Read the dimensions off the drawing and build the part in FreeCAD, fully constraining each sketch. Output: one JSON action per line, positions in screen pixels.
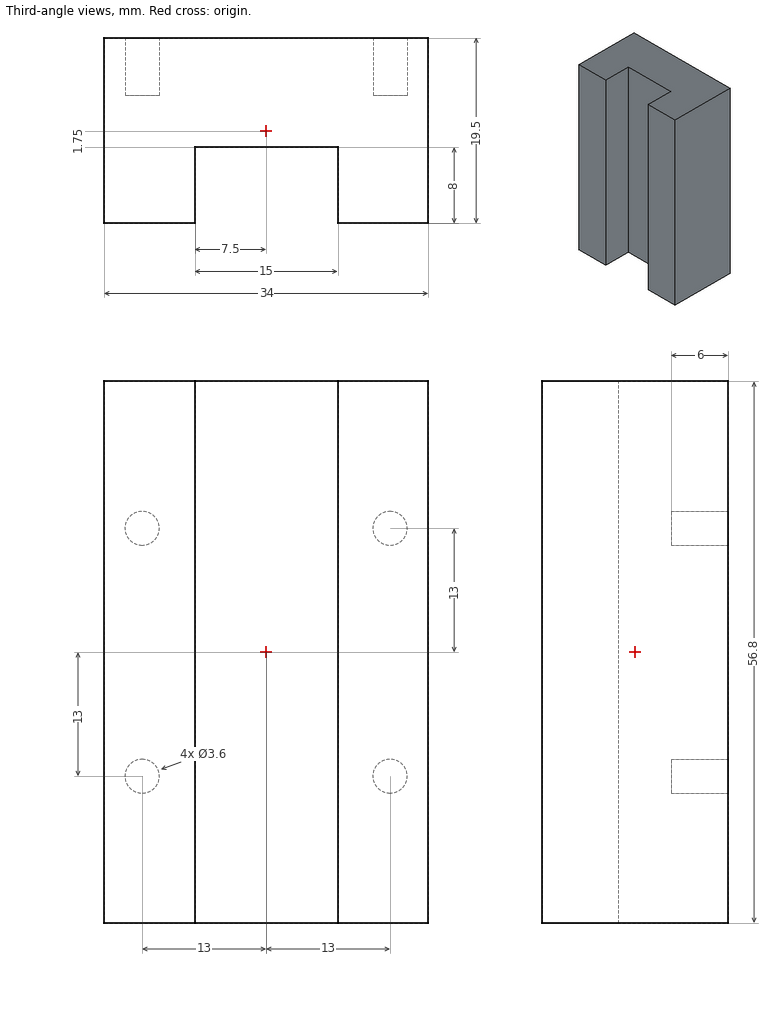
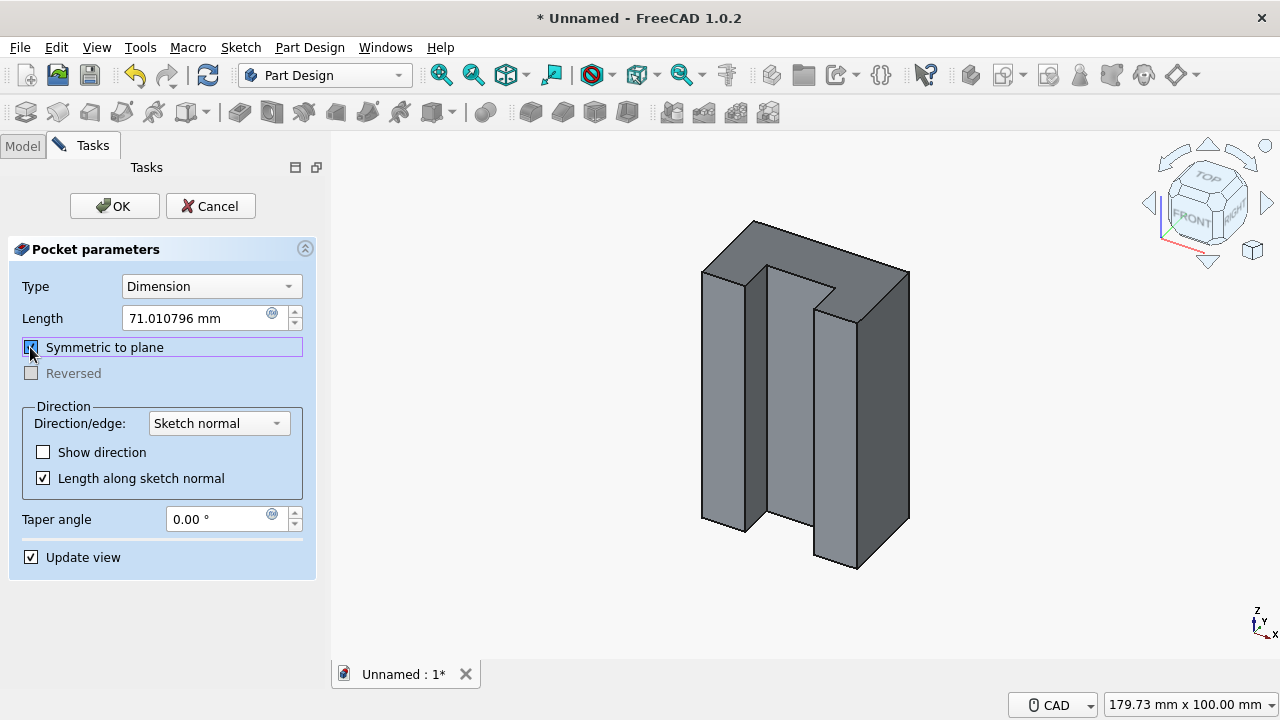
{"action": "left_click", "coordinate": [115, 206]}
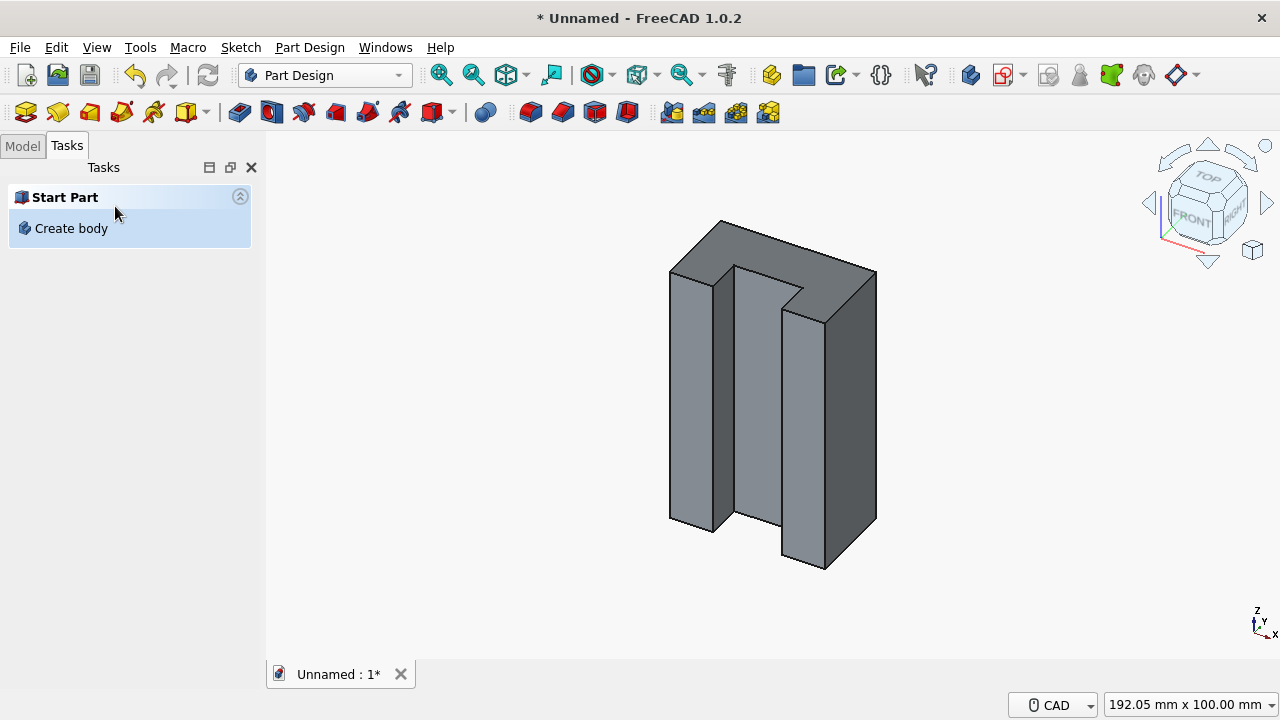
{"action": "key", "text": "4"}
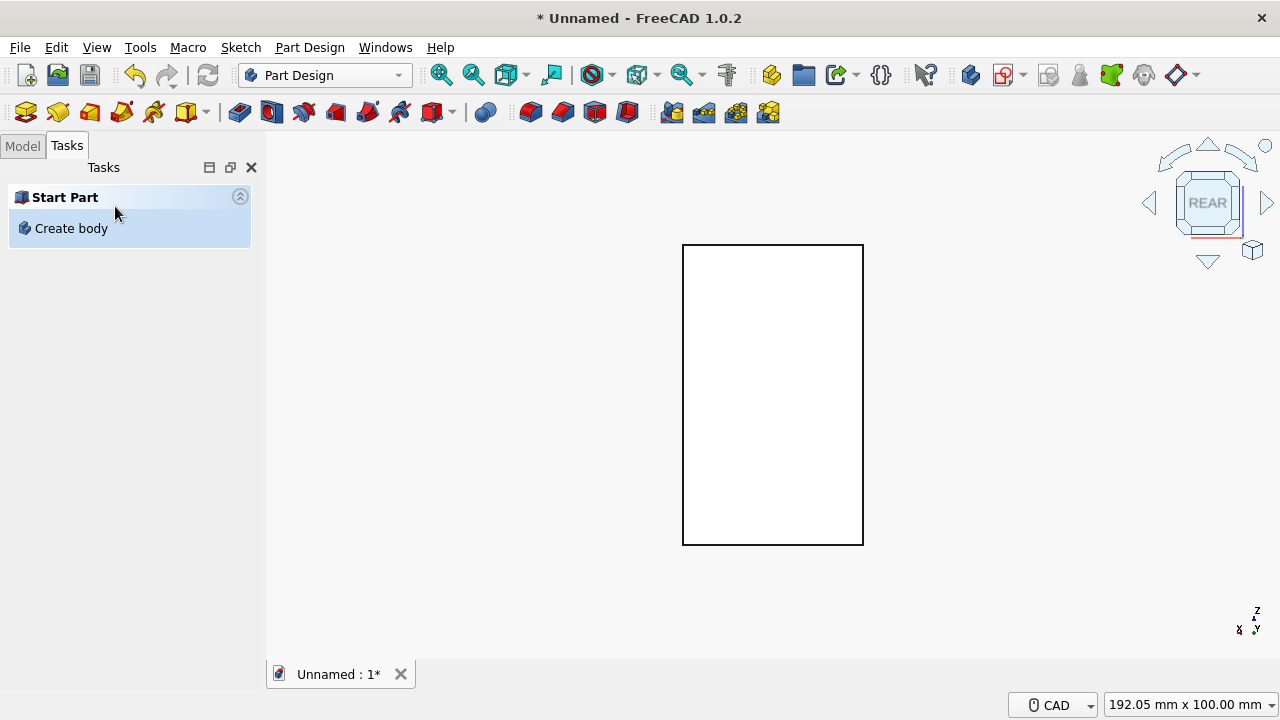
{"action": "left_click", "coordinate": [773, 351]}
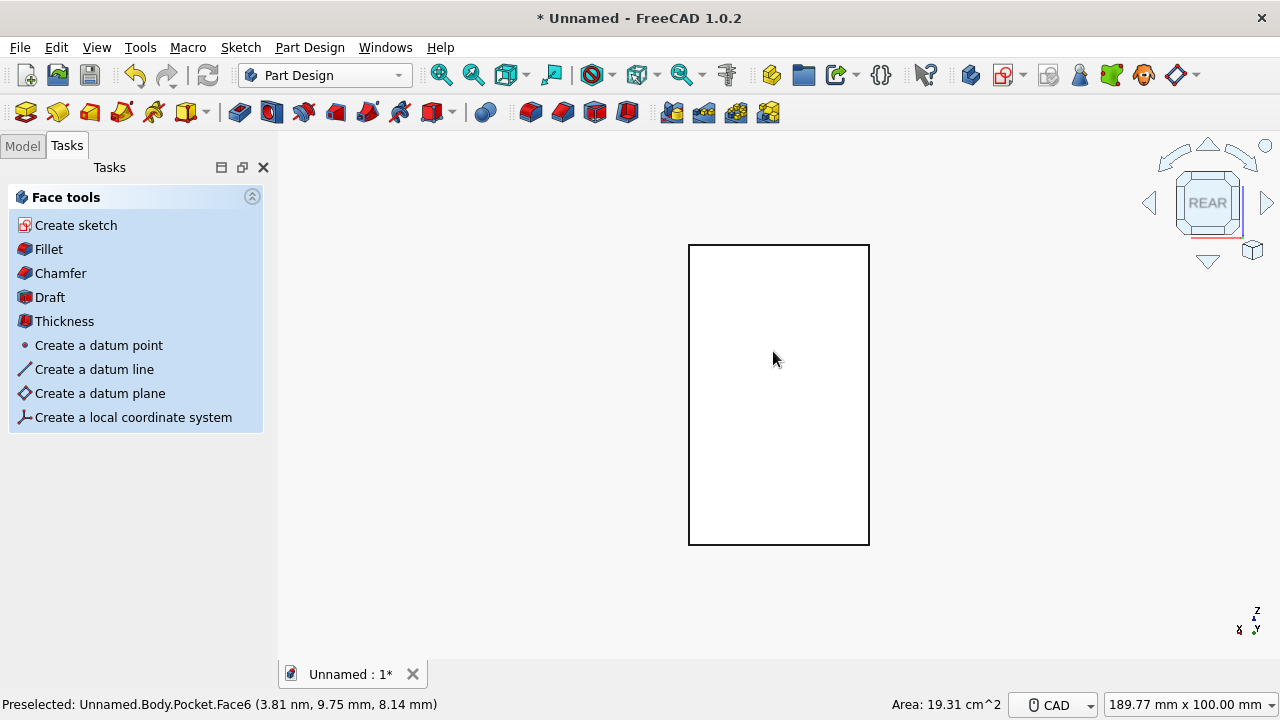
{"action": "left_click", "coordinate": [1004, 76]}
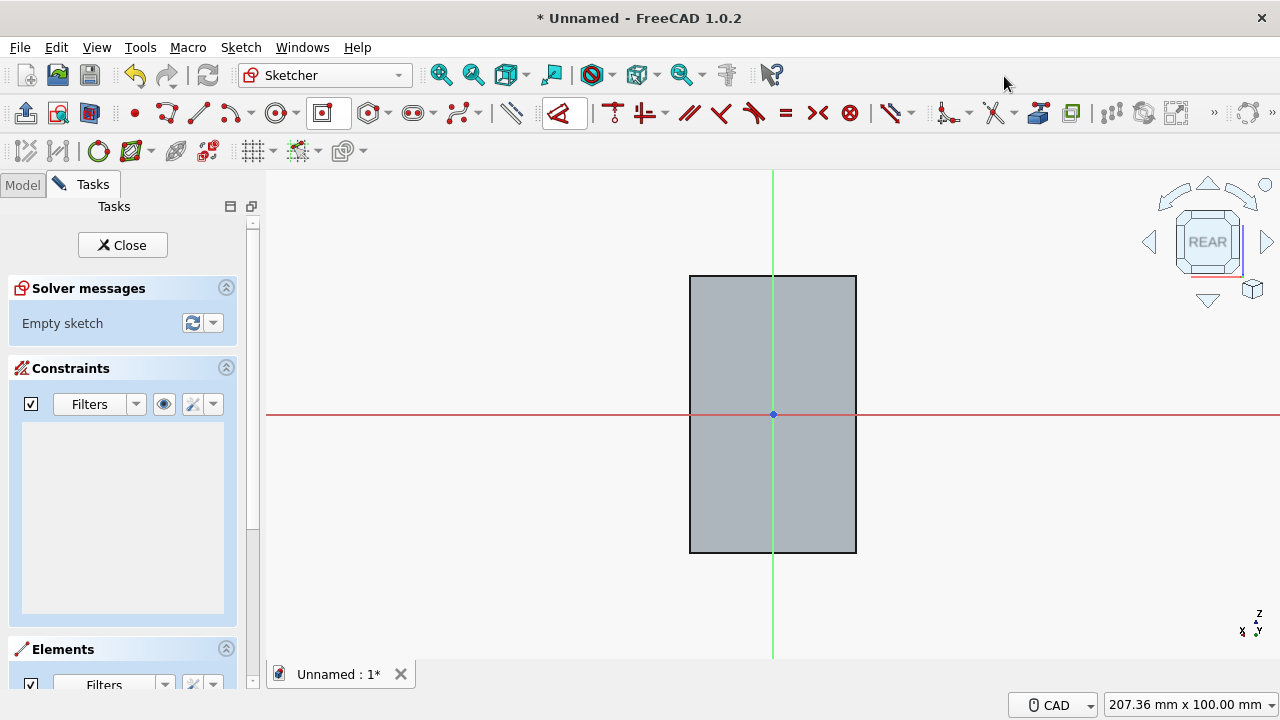
{"action": "scroll", "coordinate": [829, 414], "scroll_direction": "up", "scroll_amount": 4}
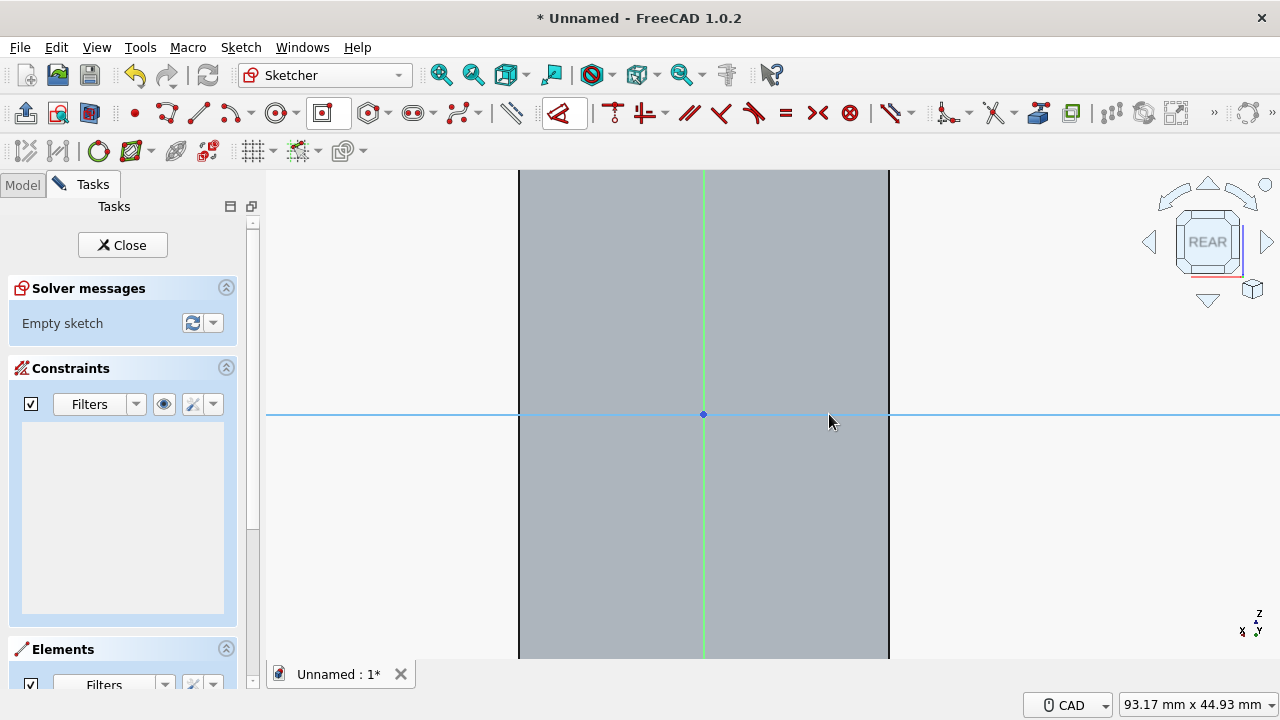
{"action": "left_click", "coordinate": [276, 114]}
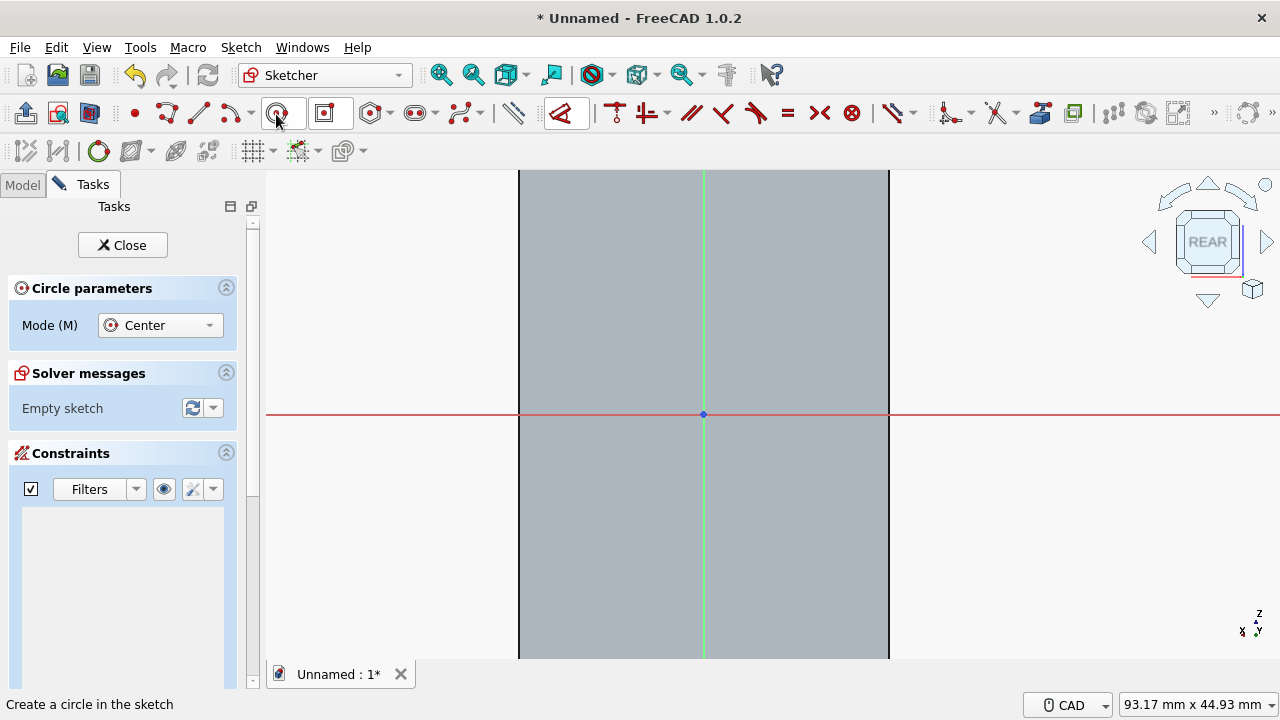
{"action": "left_click", "coordinate": [845, 556]}
{"action": "mouse_move", "coordinate": [859, 542]}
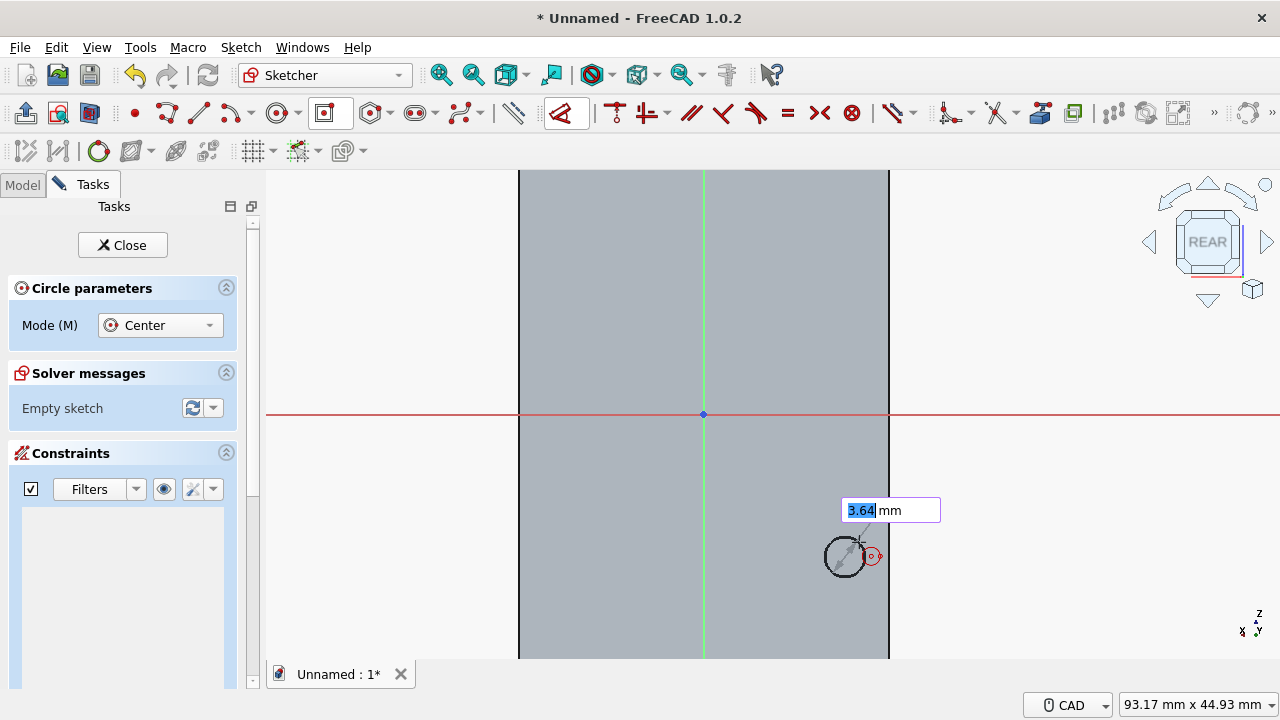
{"action": "type", "text": "3.6"}
{"action": "key", "text": "Return"}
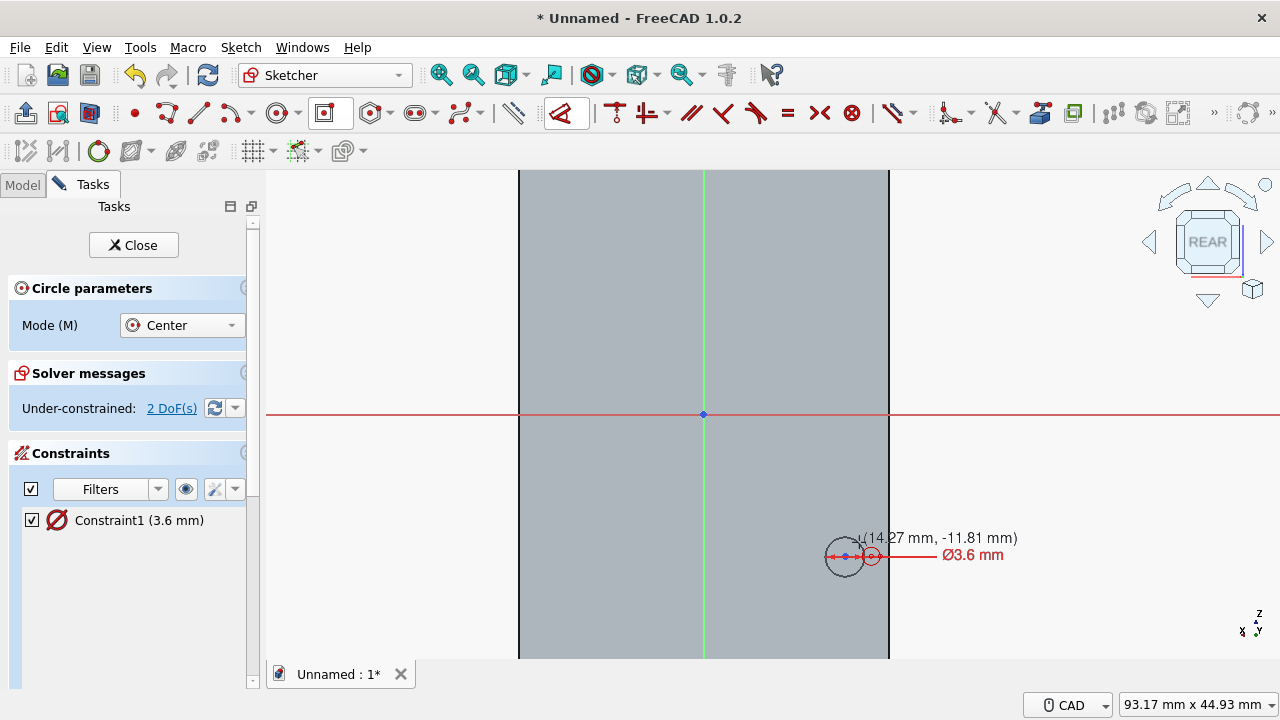
{"action": "left_click", "coordinate": [562, 556]}
{"action": "mouse_move", "coordinate": [576, 542]}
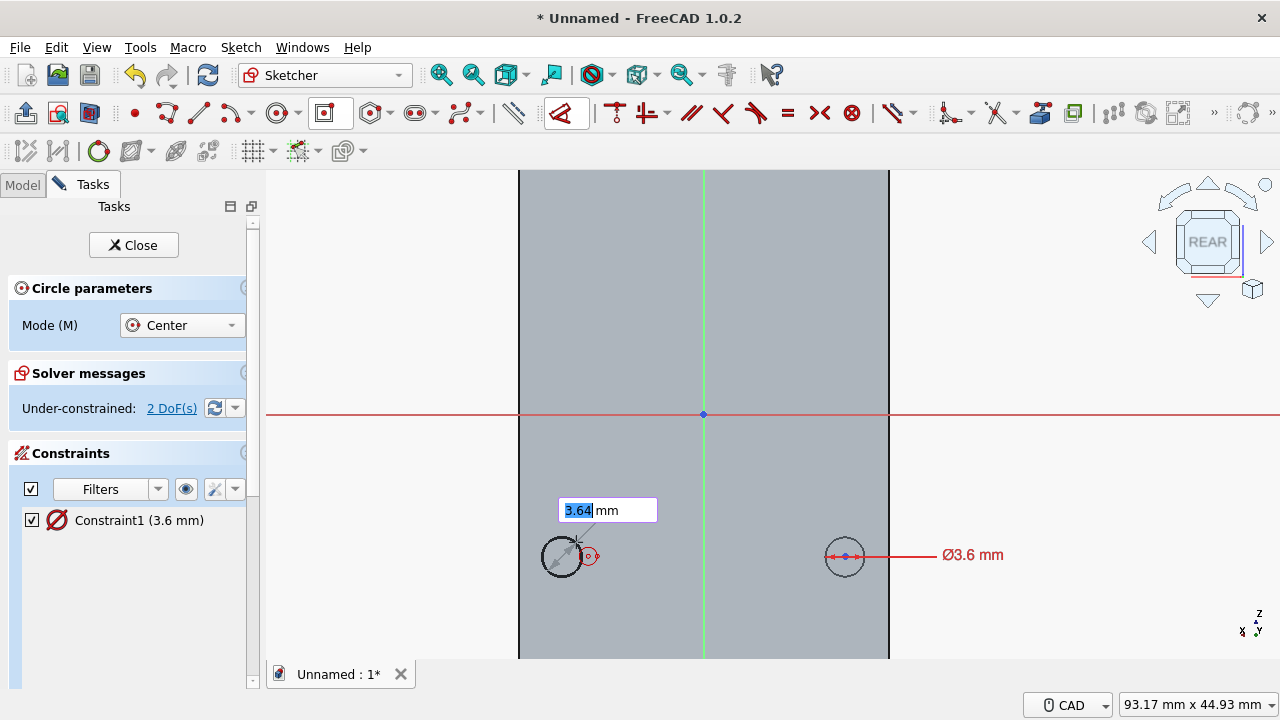
{"action": "type", "text": "3.6"}
{"action": "key", "text": "Return"}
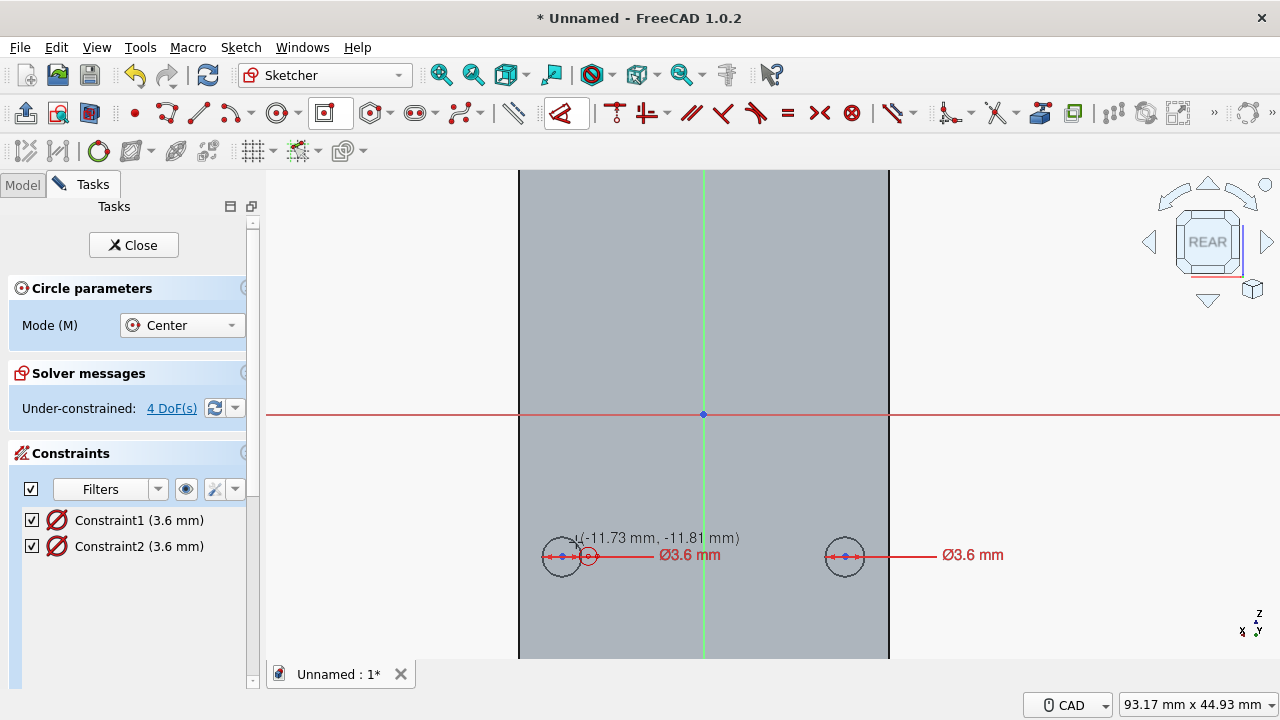
{"action": "left_click", "coordinate": [562, 273]}
{"action": "mouse_move", "coordinate": [576, 259]}